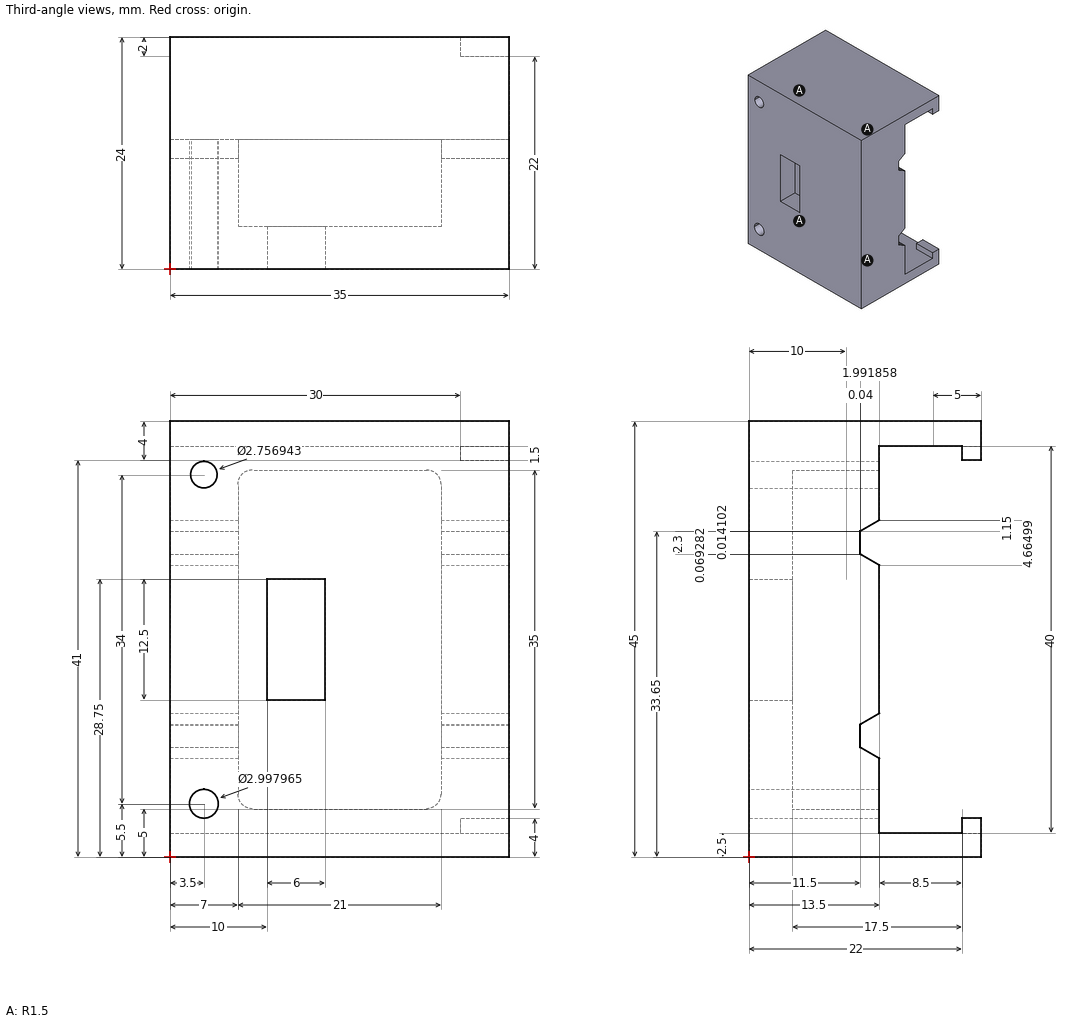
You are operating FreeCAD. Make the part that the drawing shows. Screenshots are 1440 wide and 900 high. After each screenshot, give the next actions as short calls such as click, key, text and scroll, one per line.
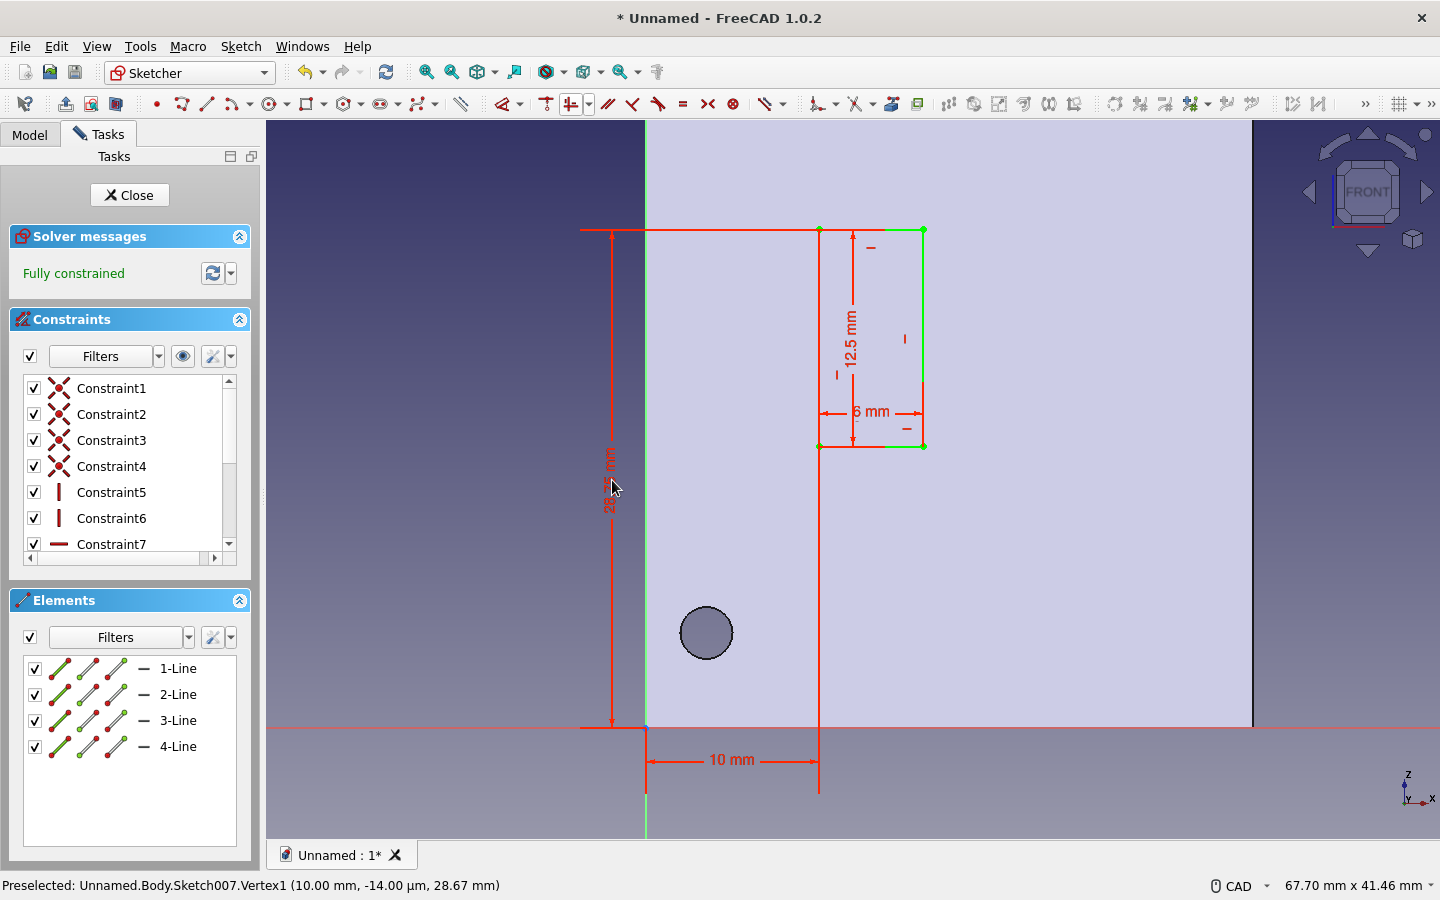
click(130, 195)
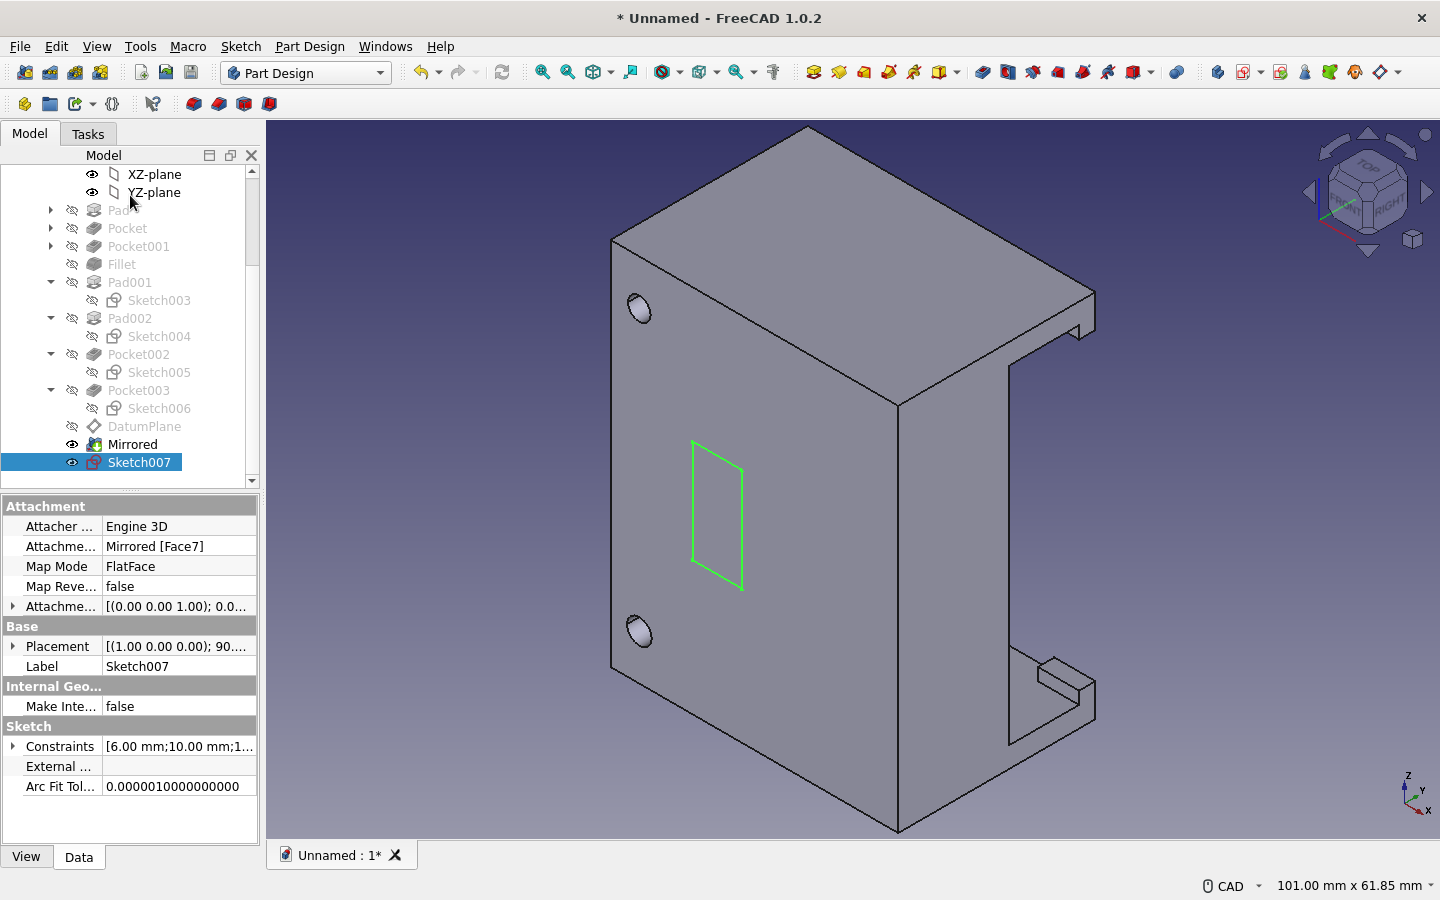
click(983, 72)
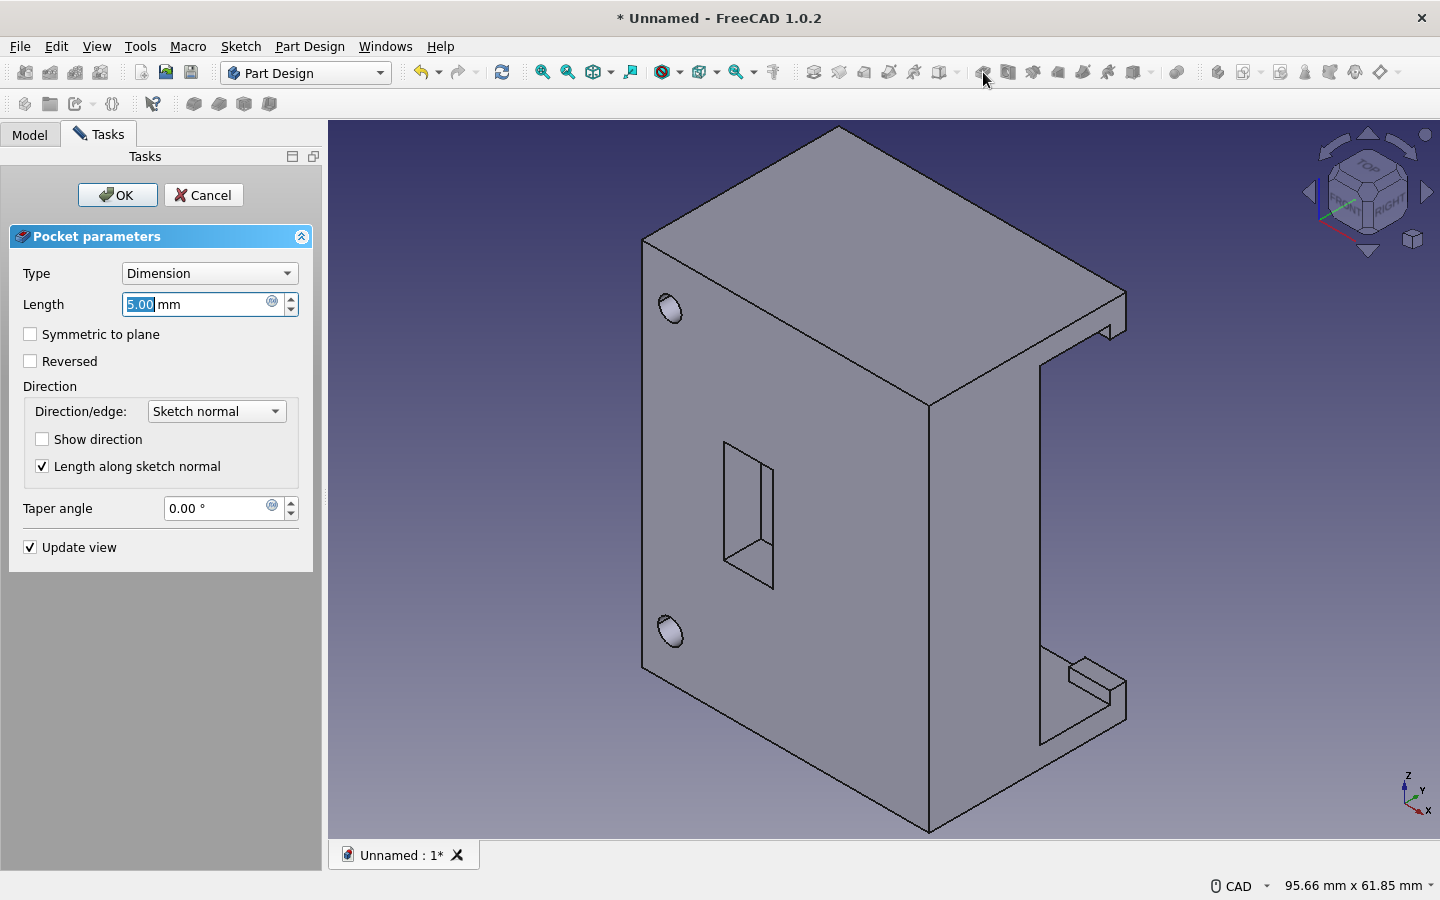
text(10)
key(Tab)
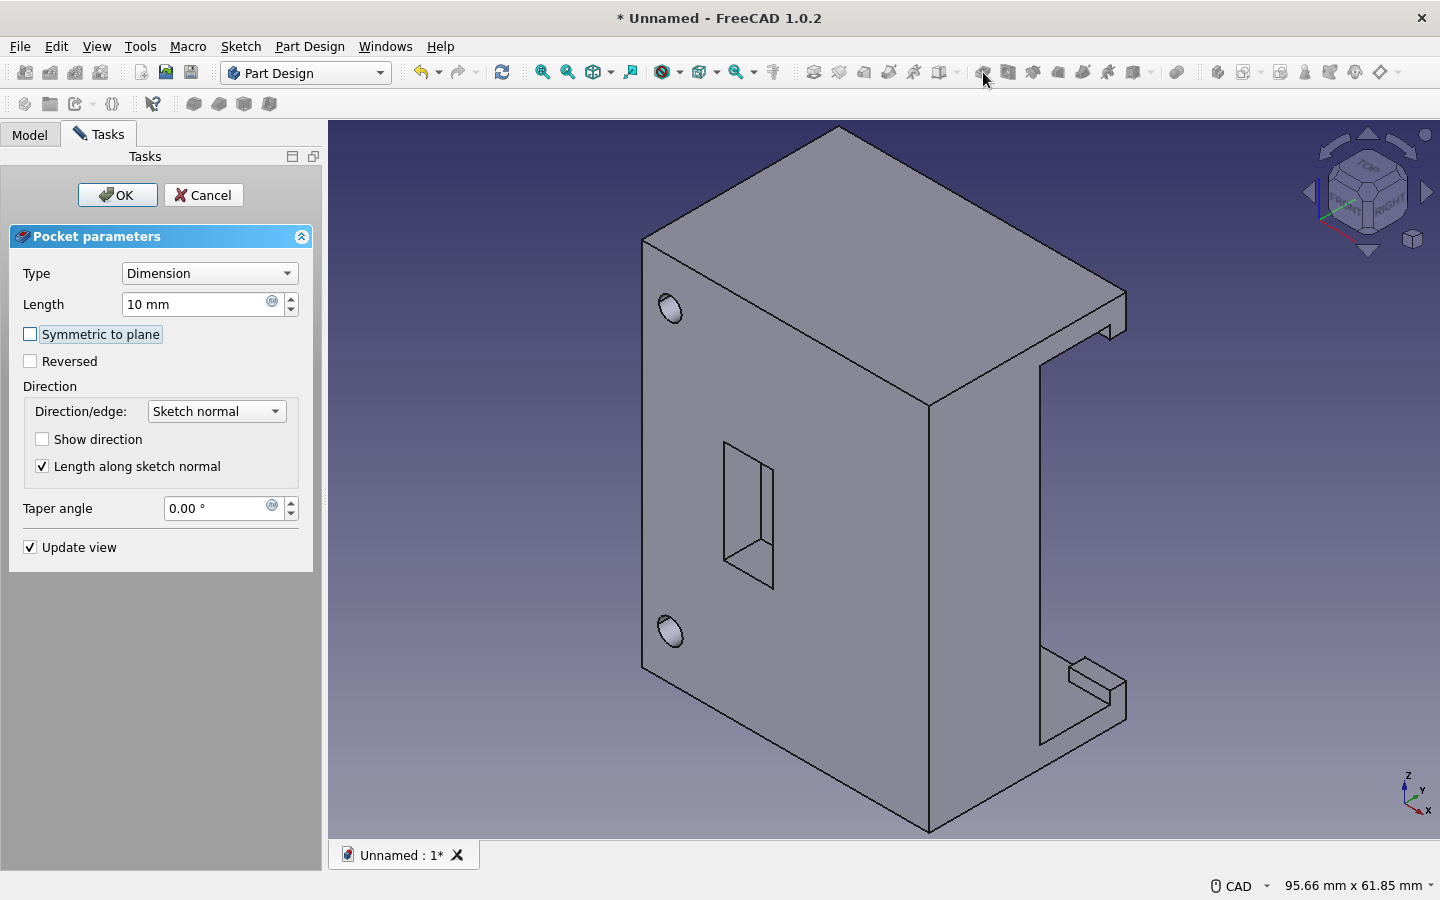
click(118, 195)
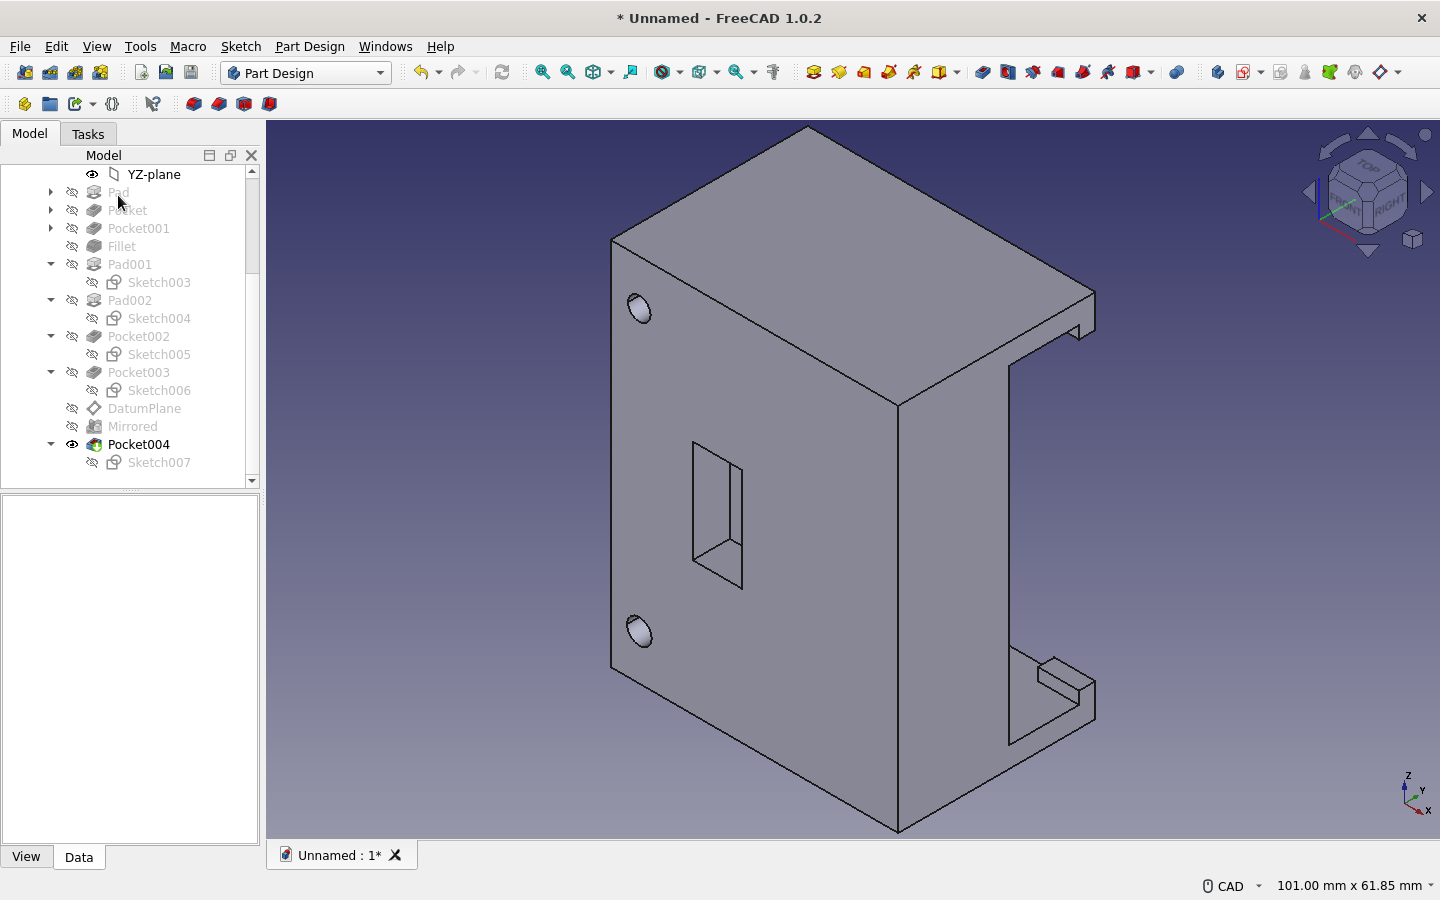
click(940, 472)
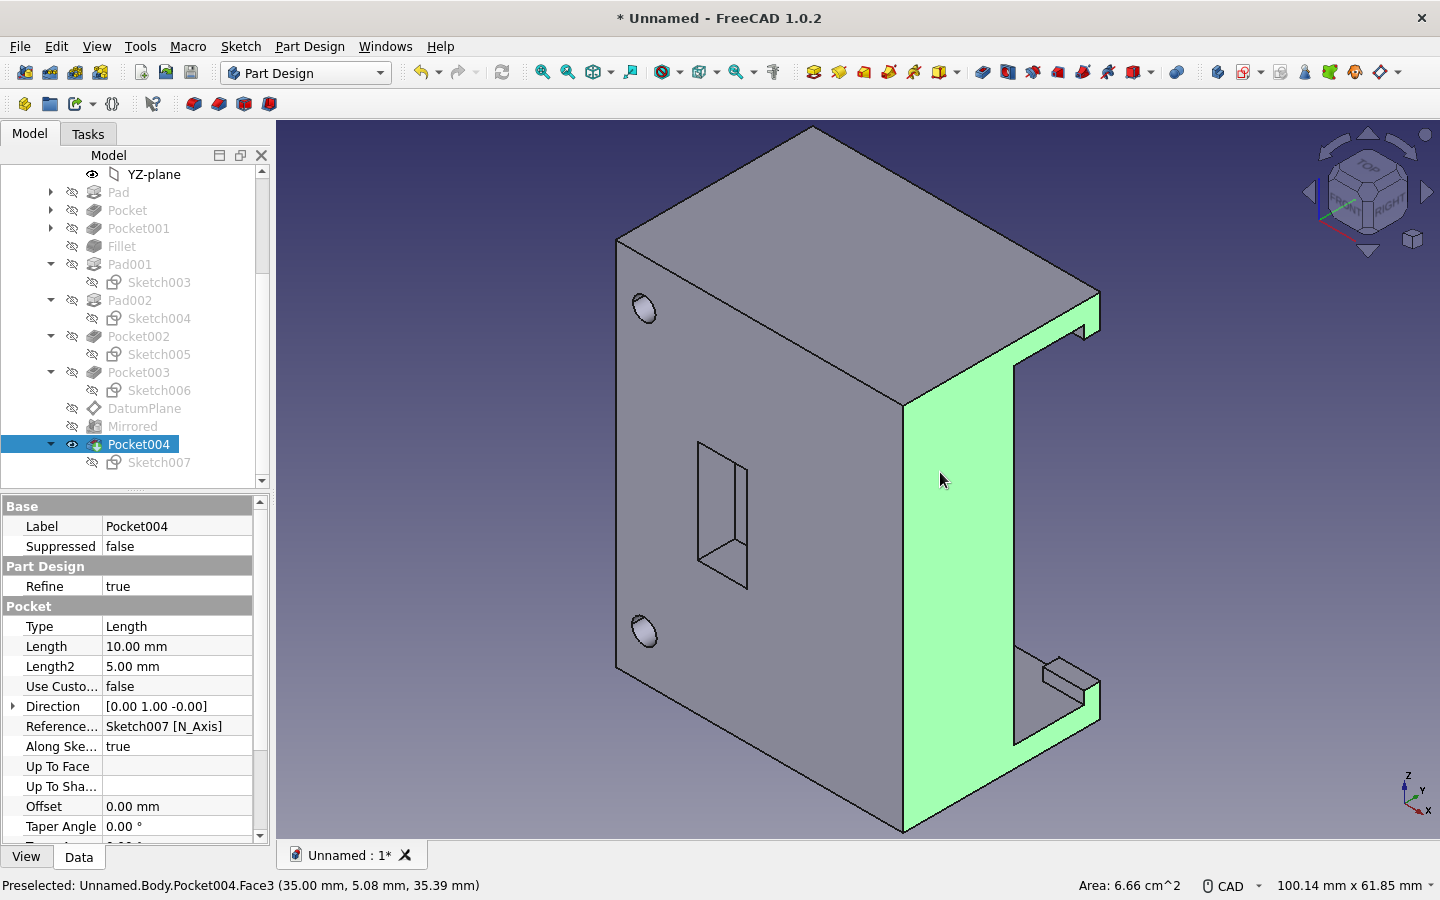
click(1242, 72)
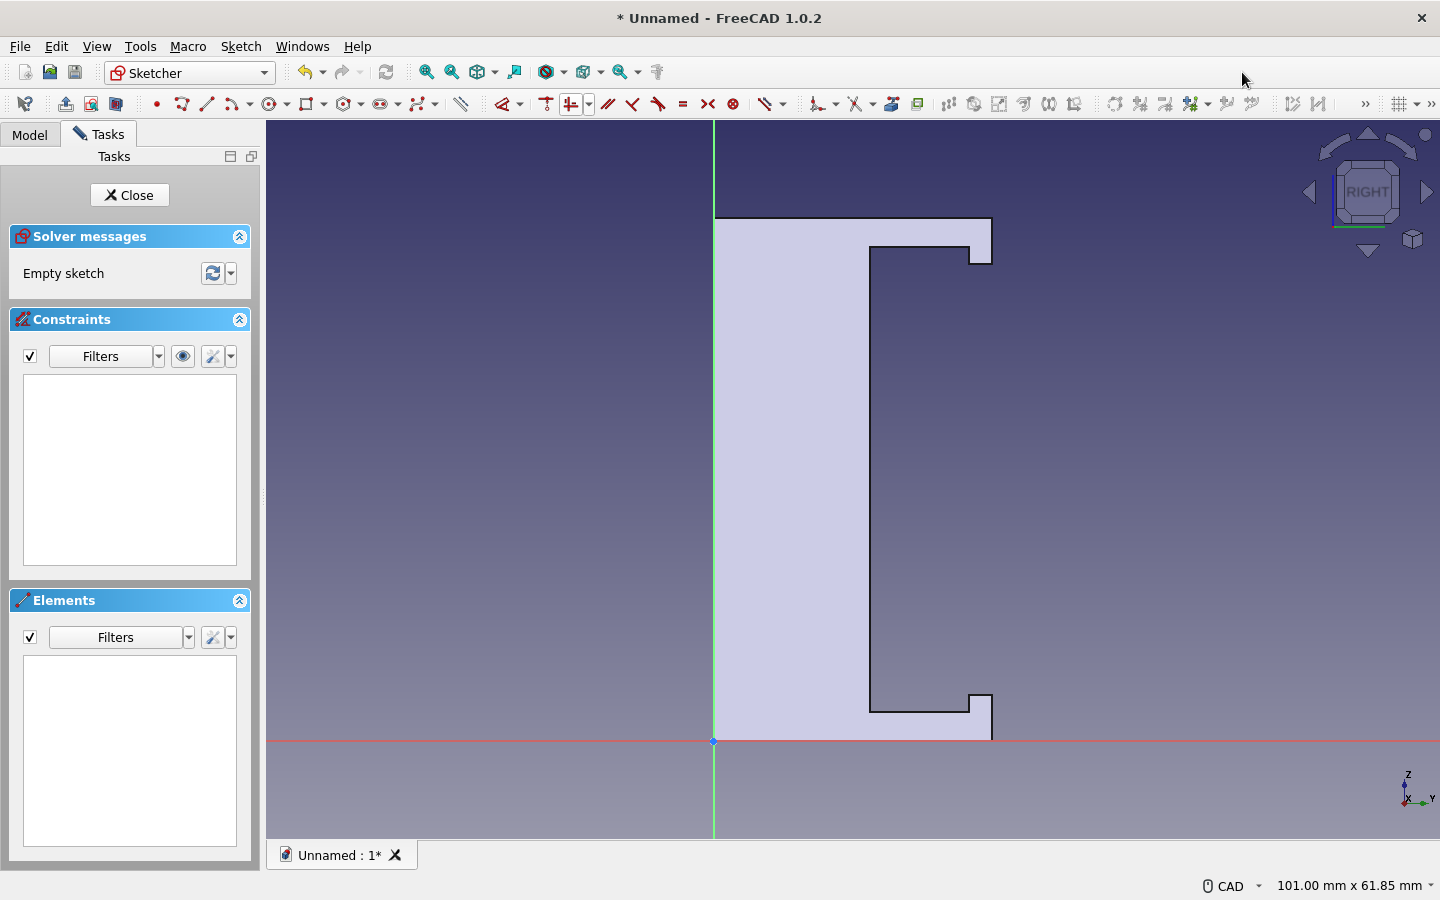
scroll(868, 349, up, 11)